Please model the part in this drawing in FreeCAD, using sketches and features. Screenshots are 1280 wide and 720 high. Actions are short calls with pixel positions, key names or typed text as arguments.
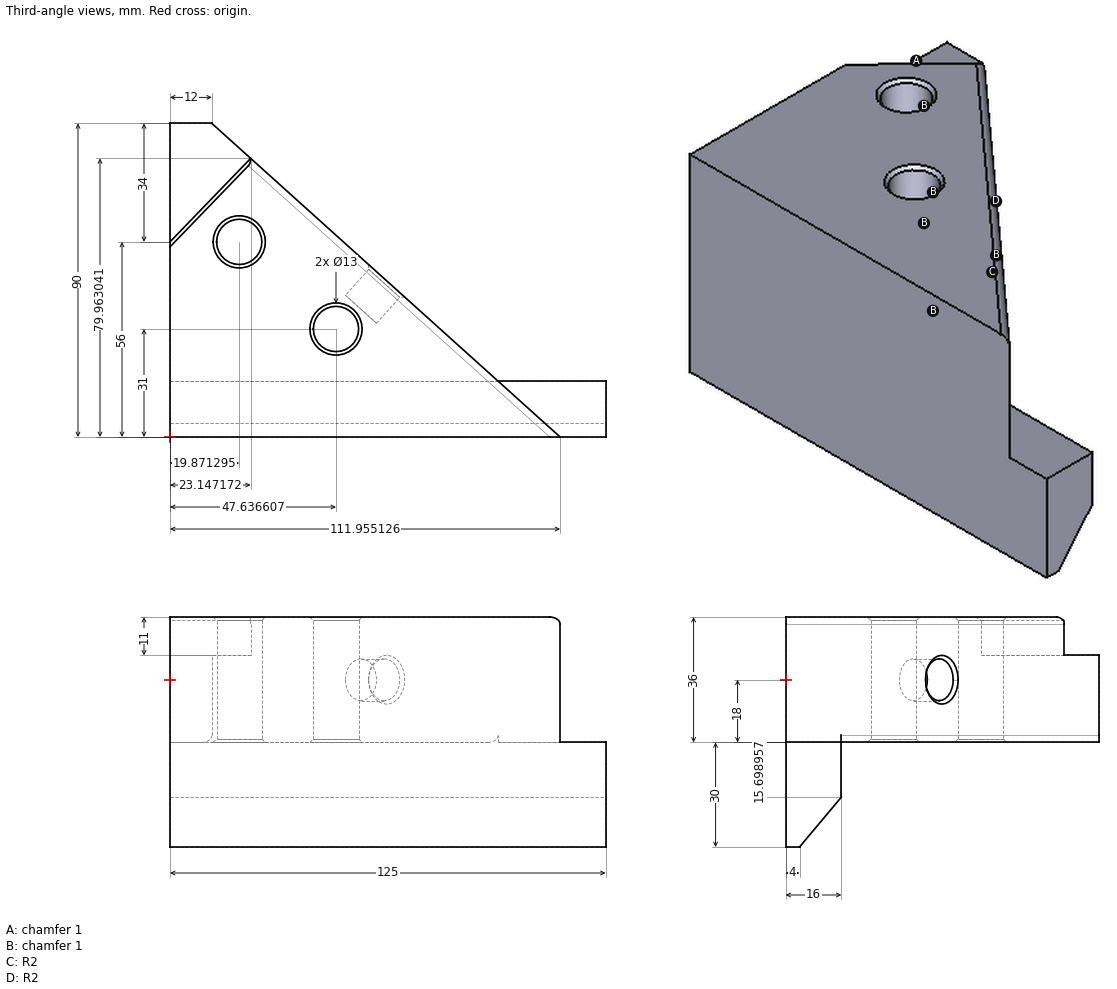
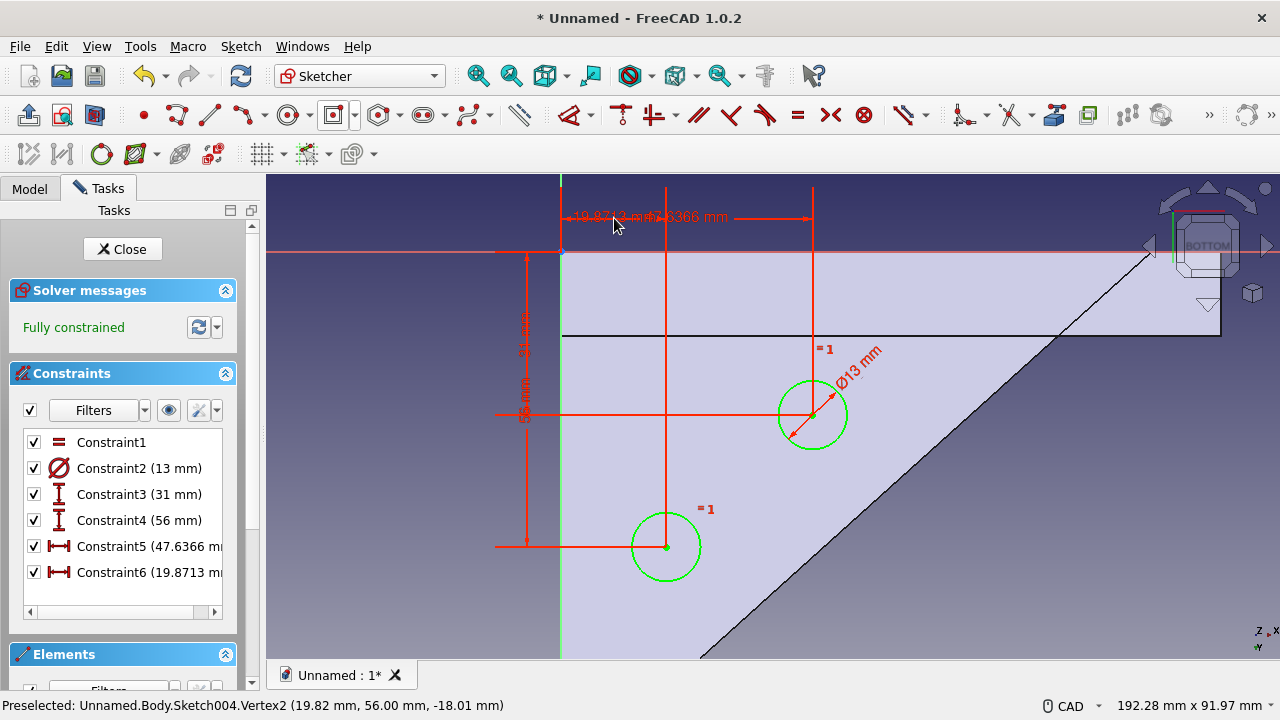
click(123, 249)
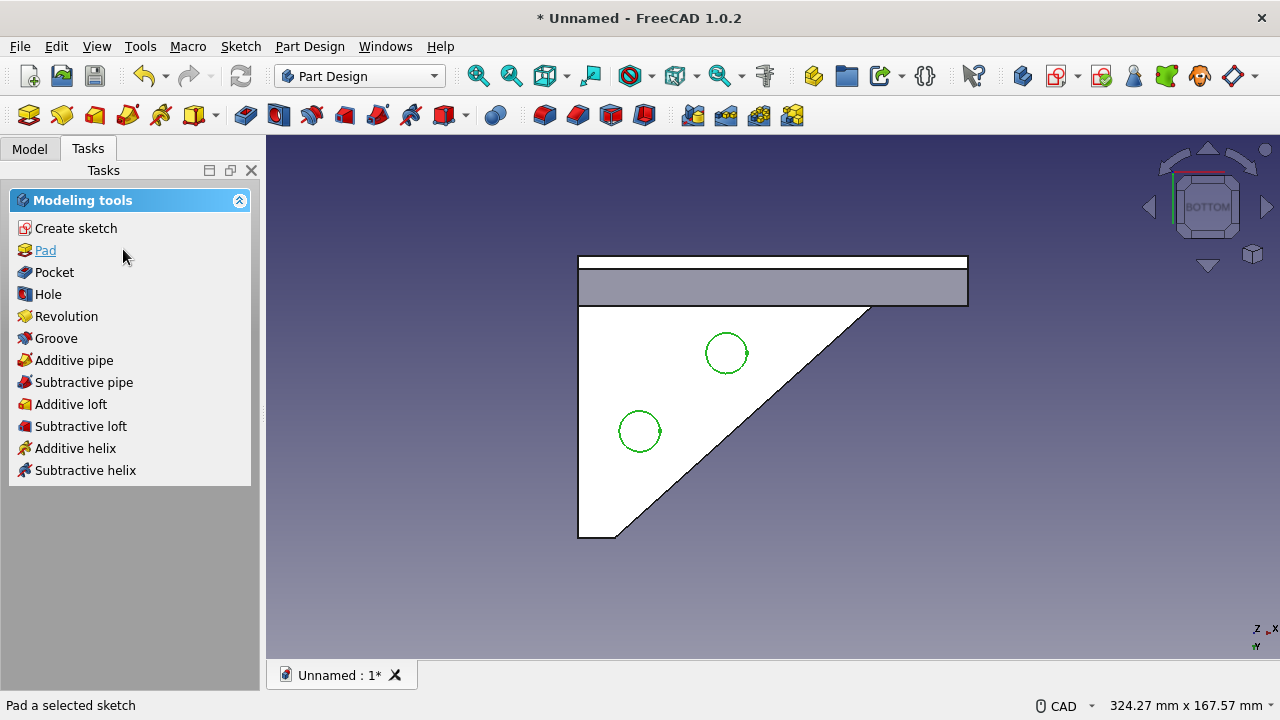
click(246, 116)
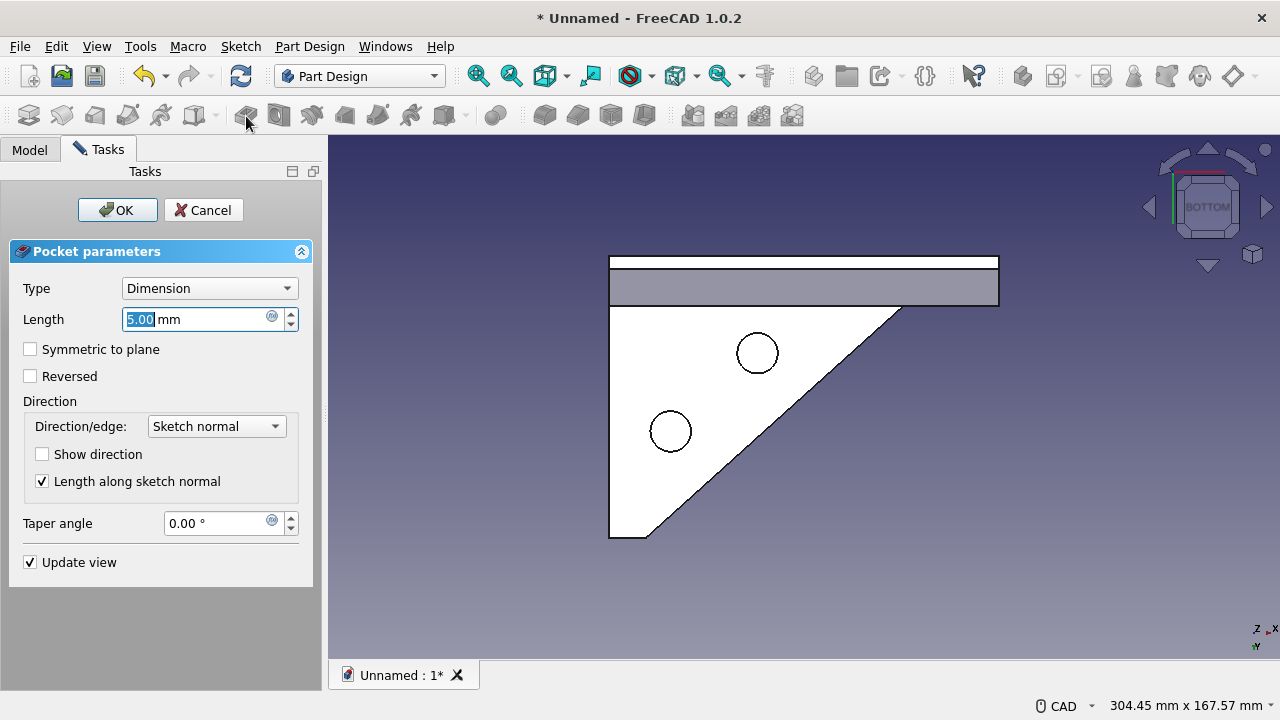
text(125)
key(Tab)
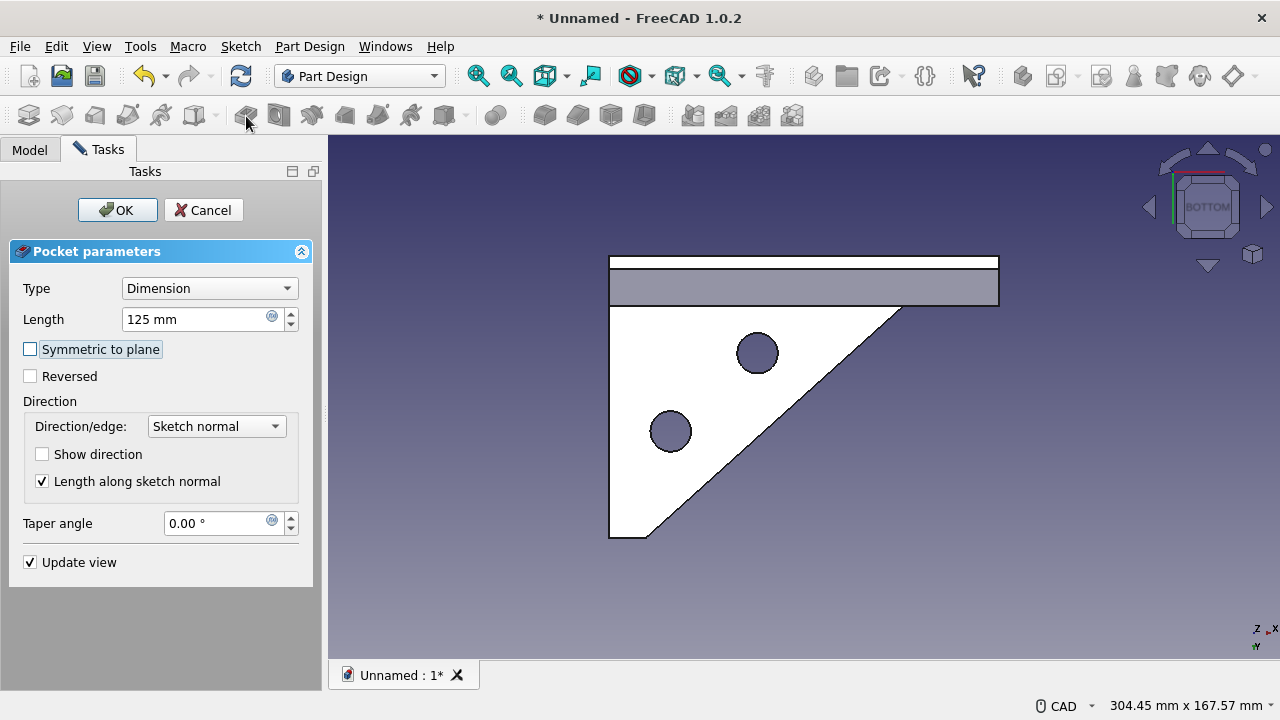
click(118, 210)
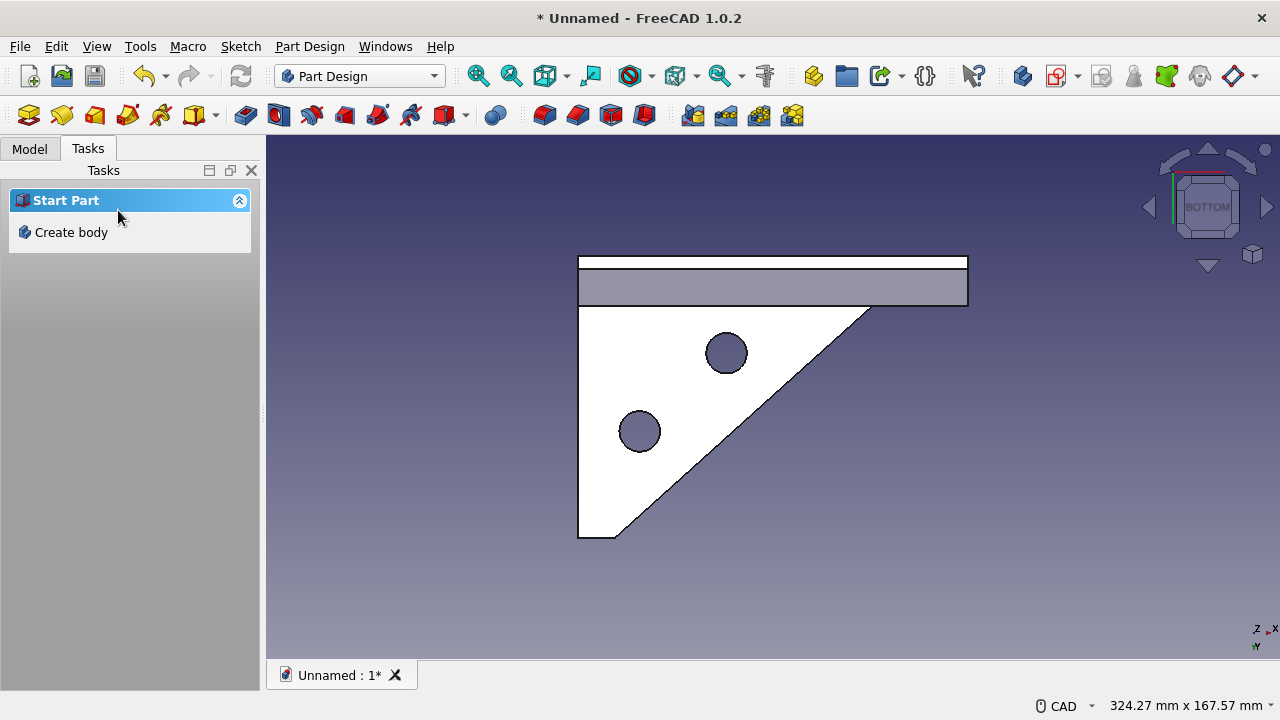
key(0)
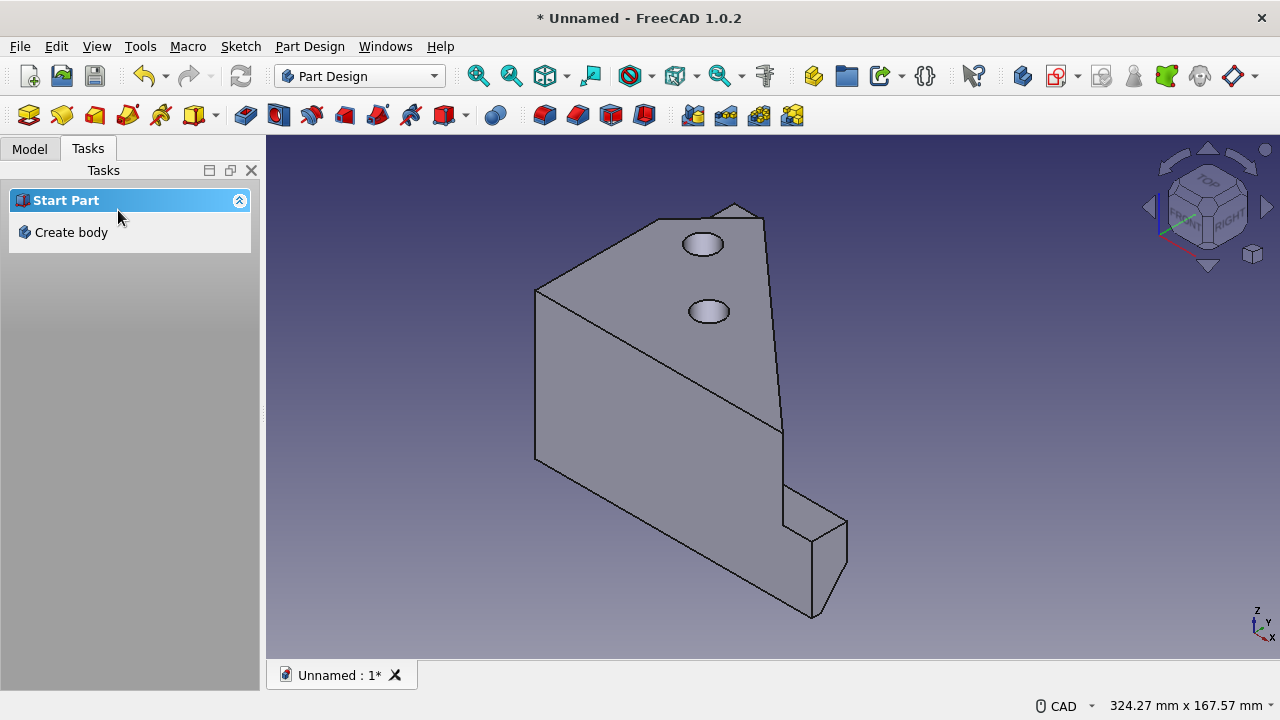
key(2)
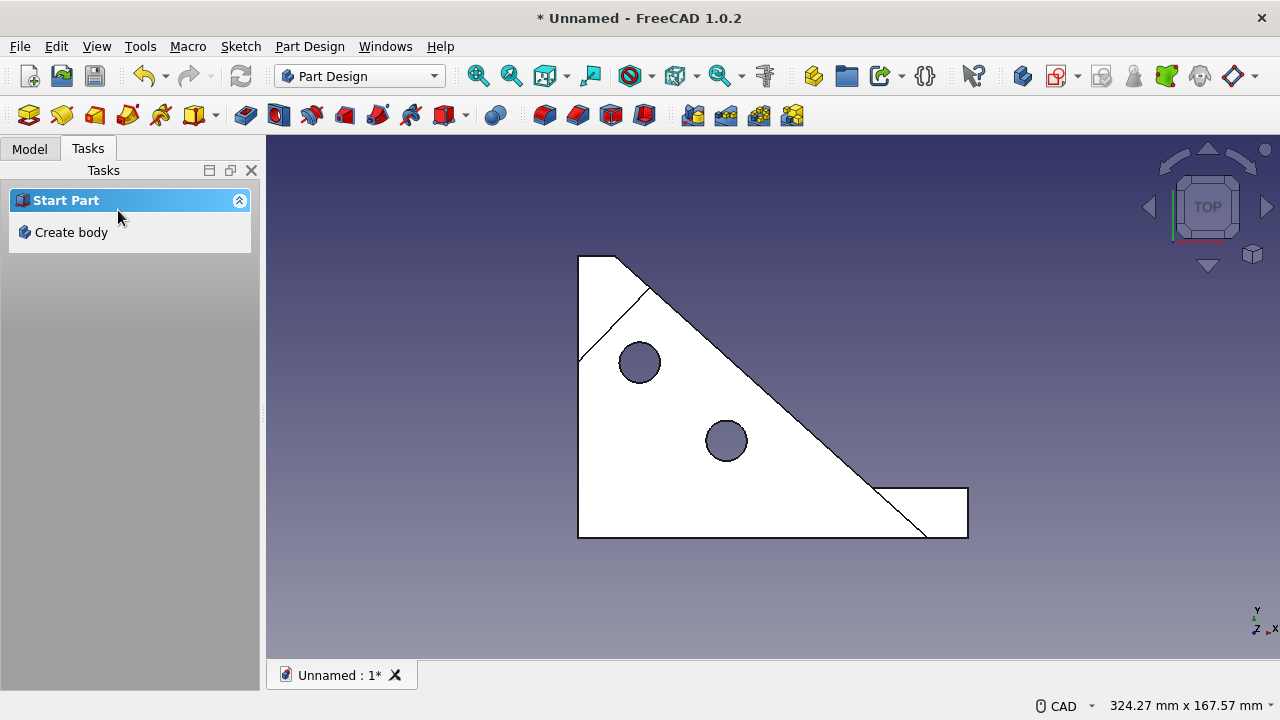
click(614, 324)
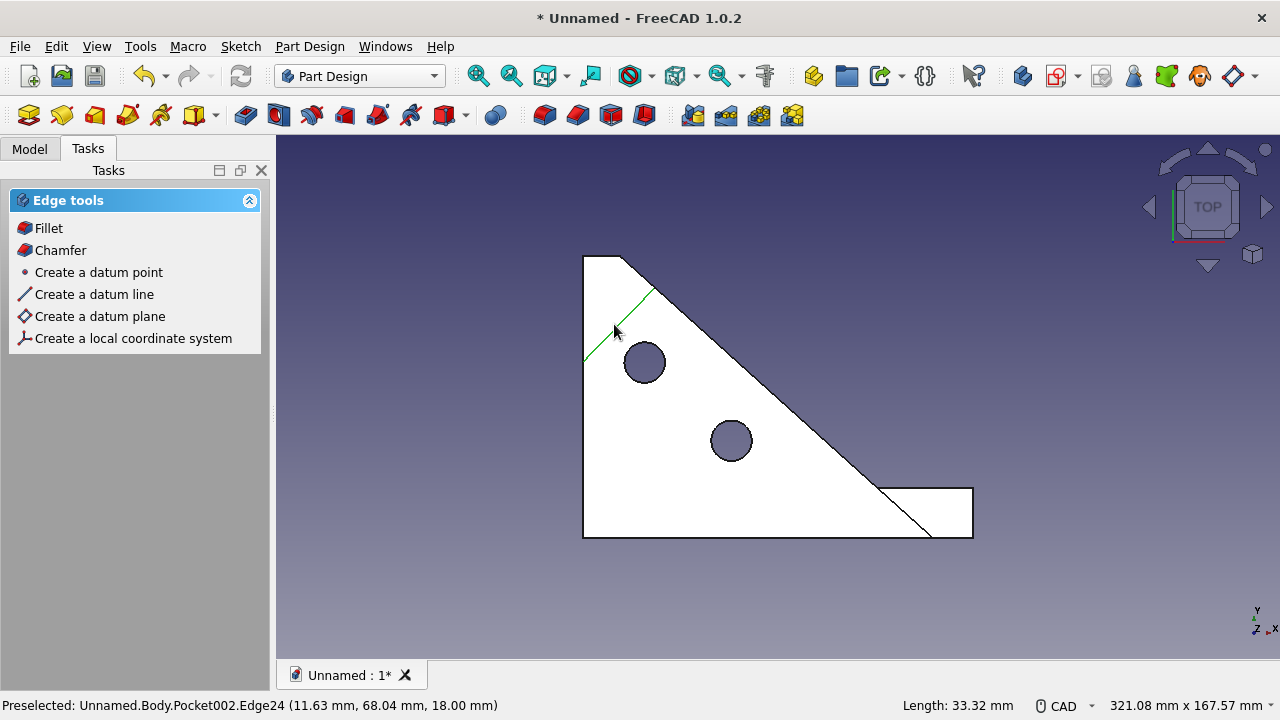
click(578, 116)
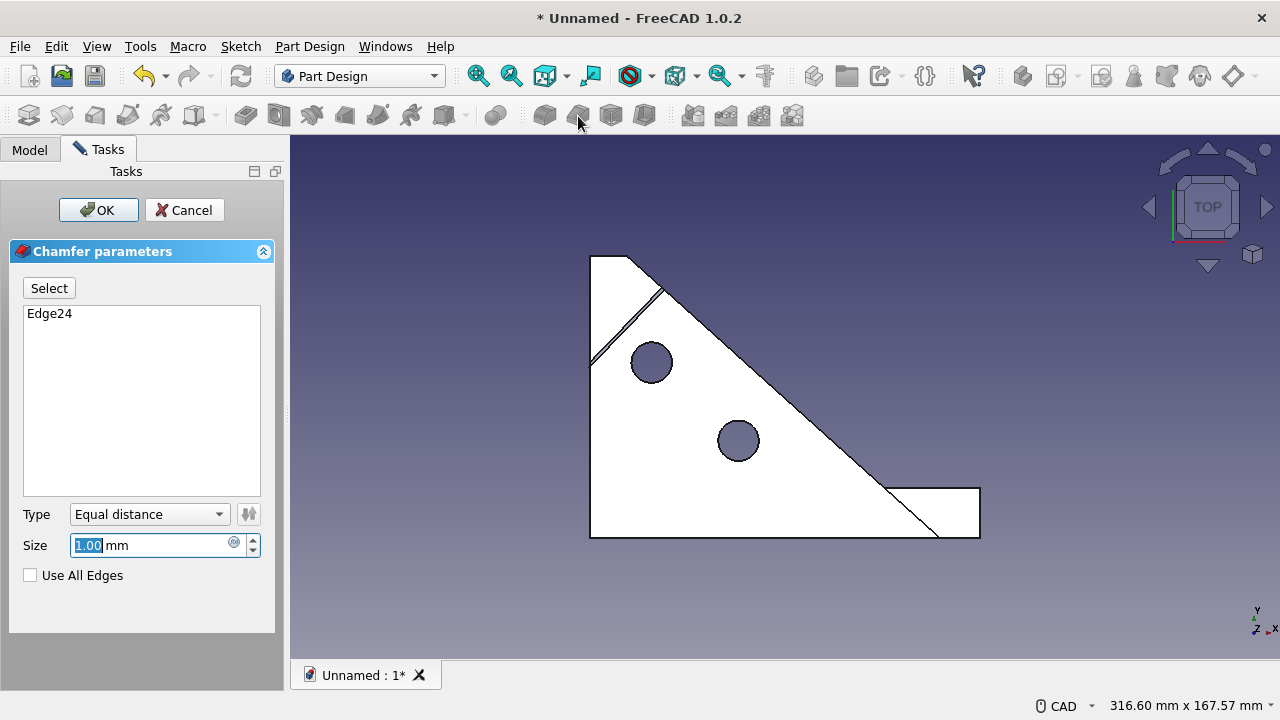
text(1)
key(Tab)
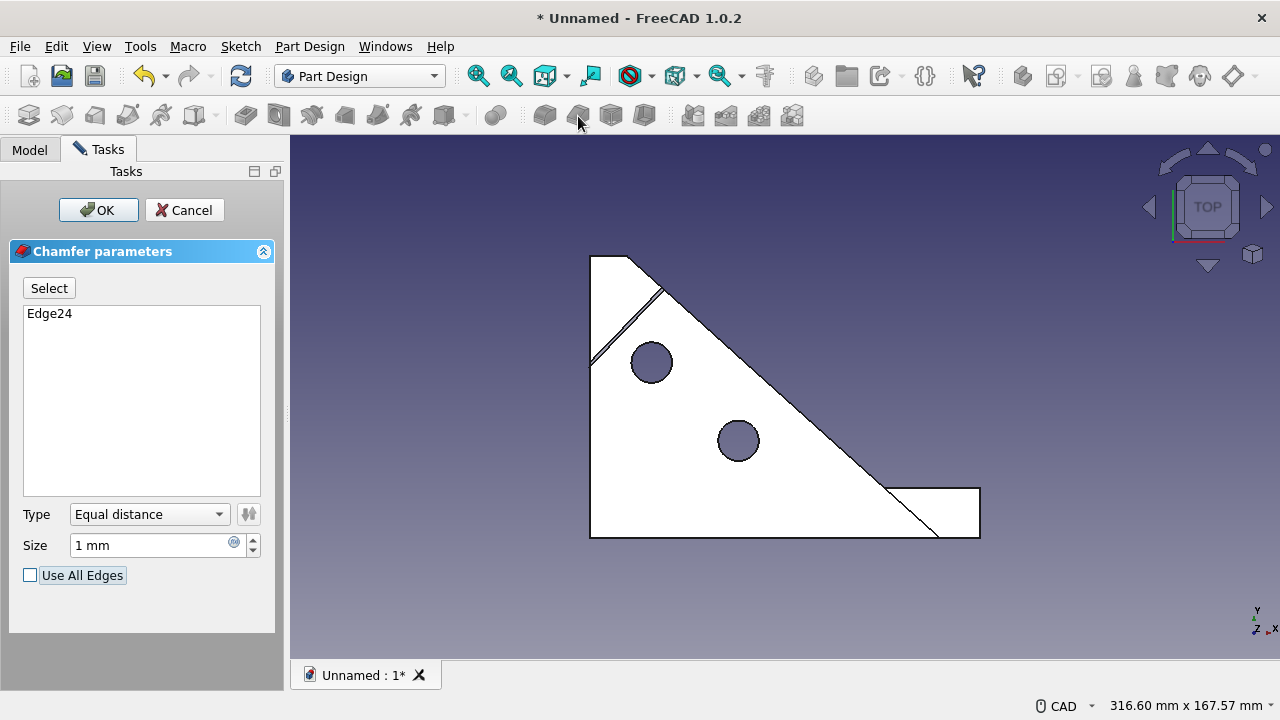
click(99, 210)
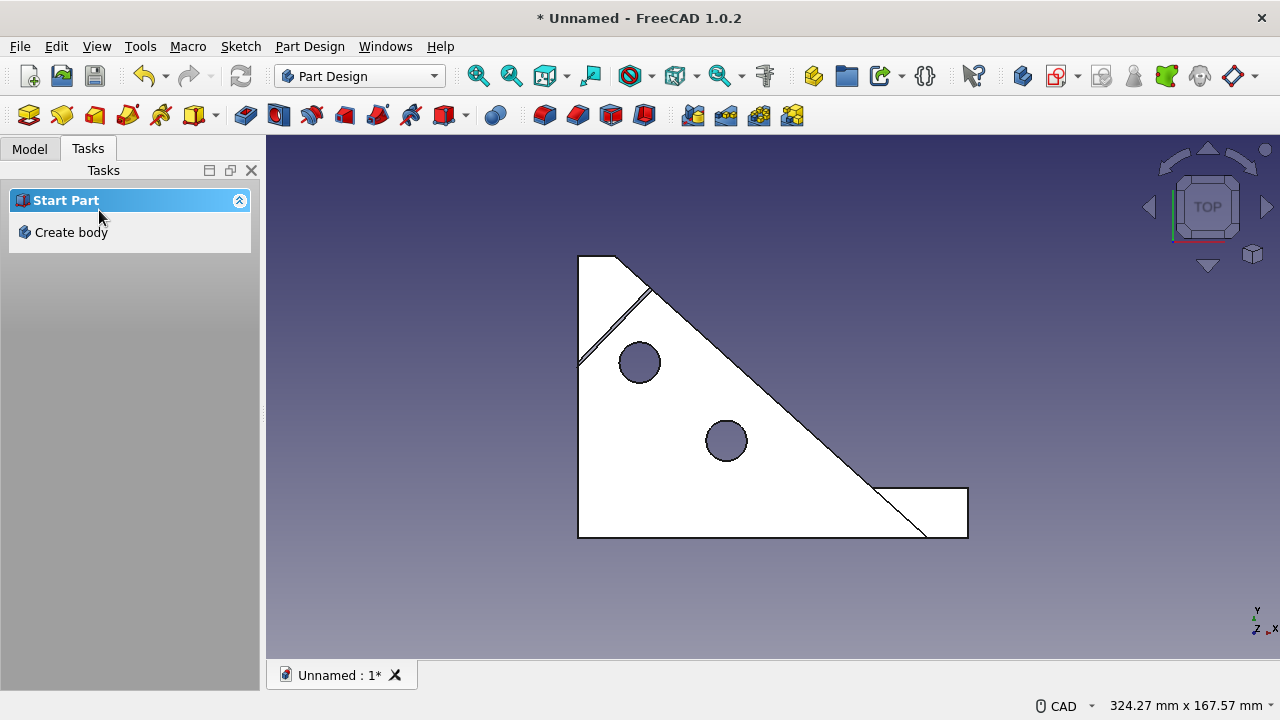
click(706, 440)